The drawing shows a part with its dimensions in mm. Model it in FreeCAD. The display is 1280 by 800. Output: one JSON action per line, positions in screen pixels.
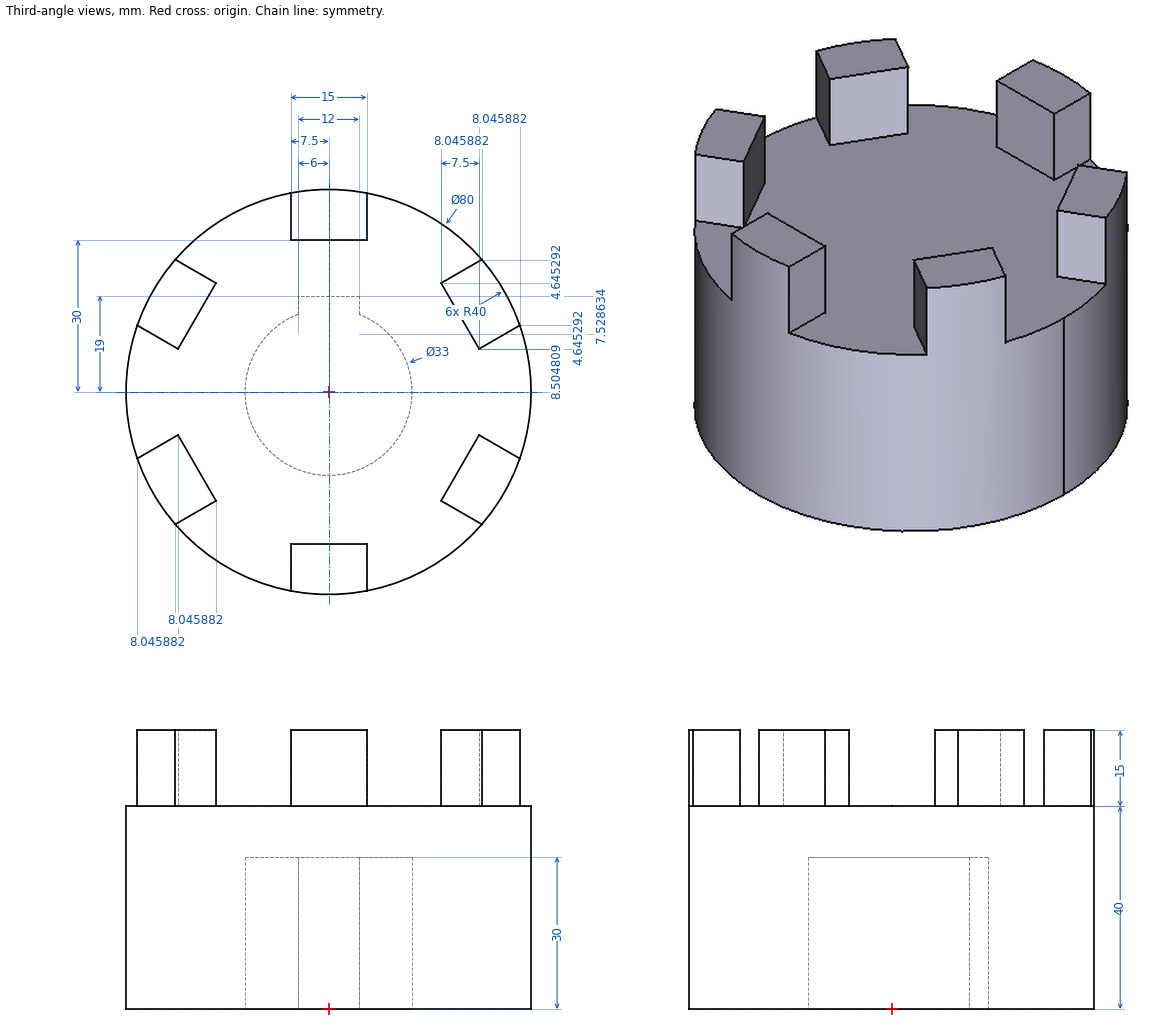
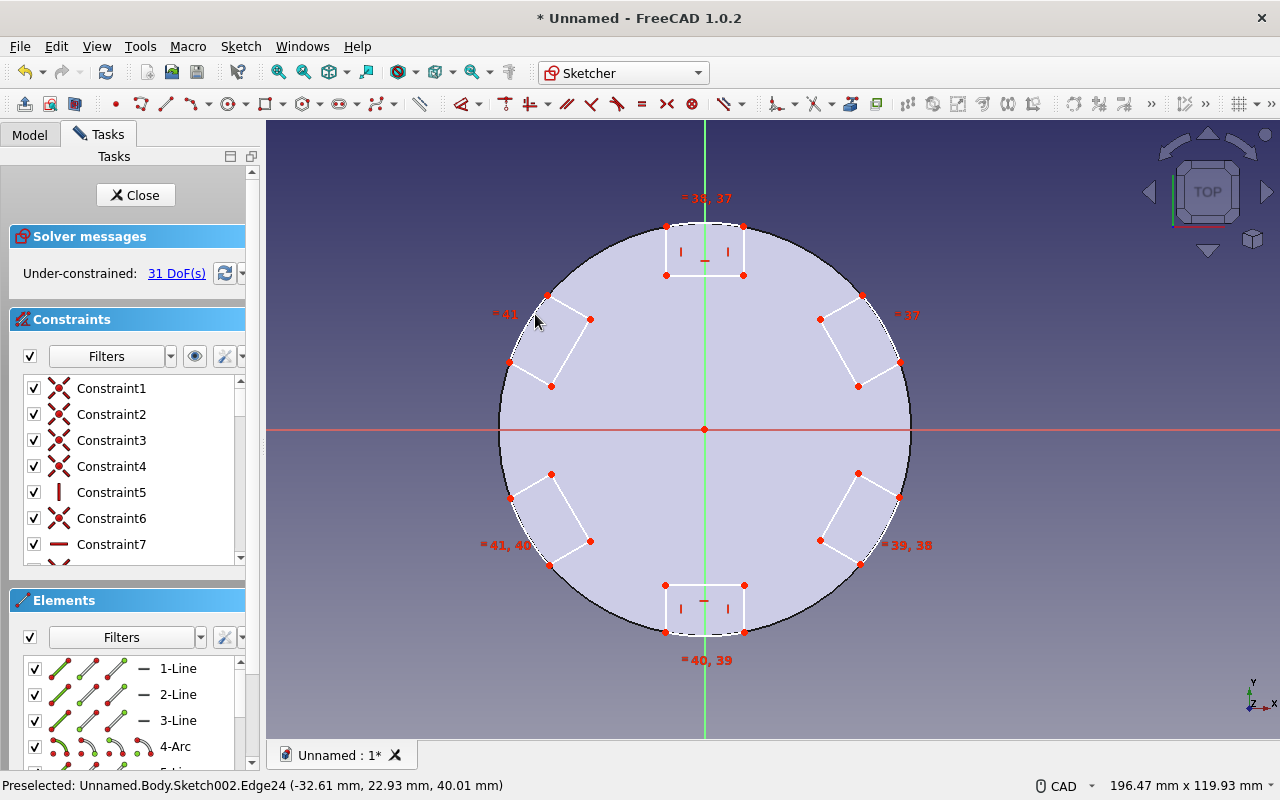
{"action": "left_click", "coordinate": [858, 387]}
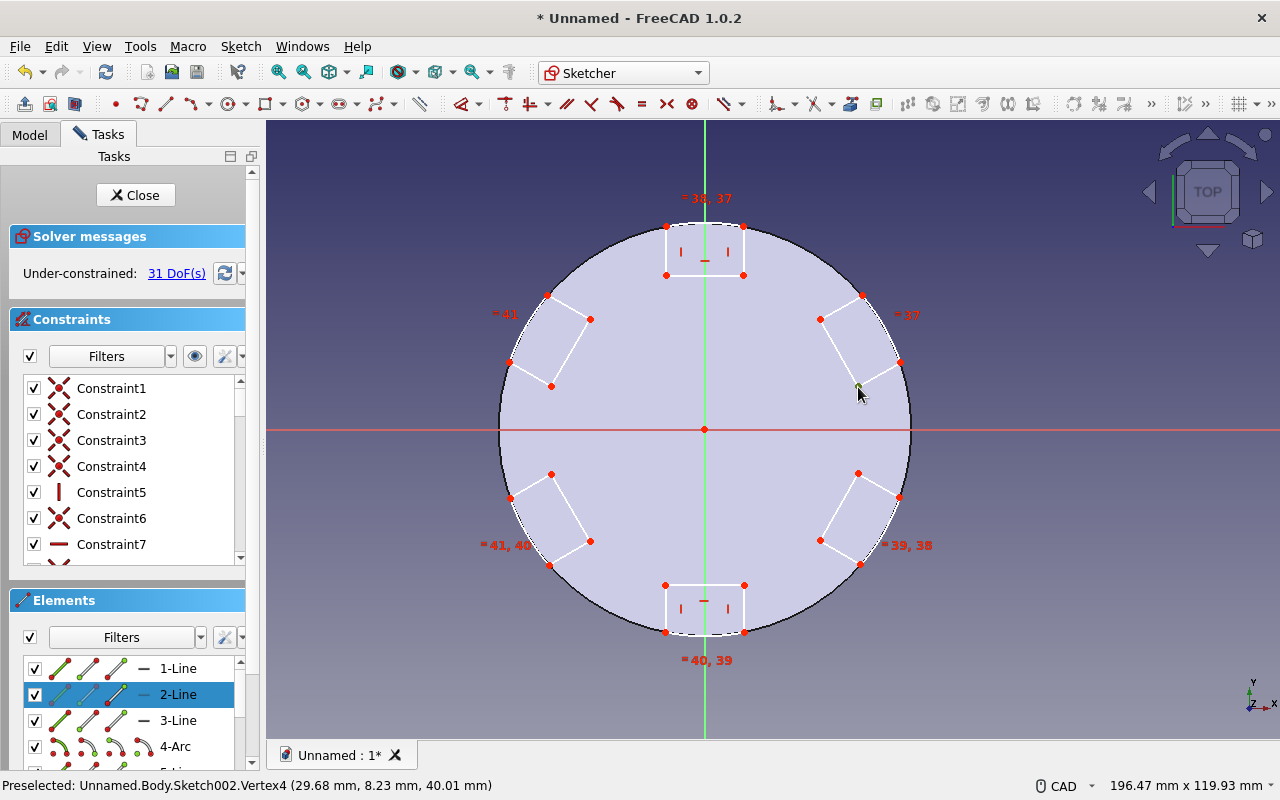
{"action": "left_click", "coordinate": [858, 474]}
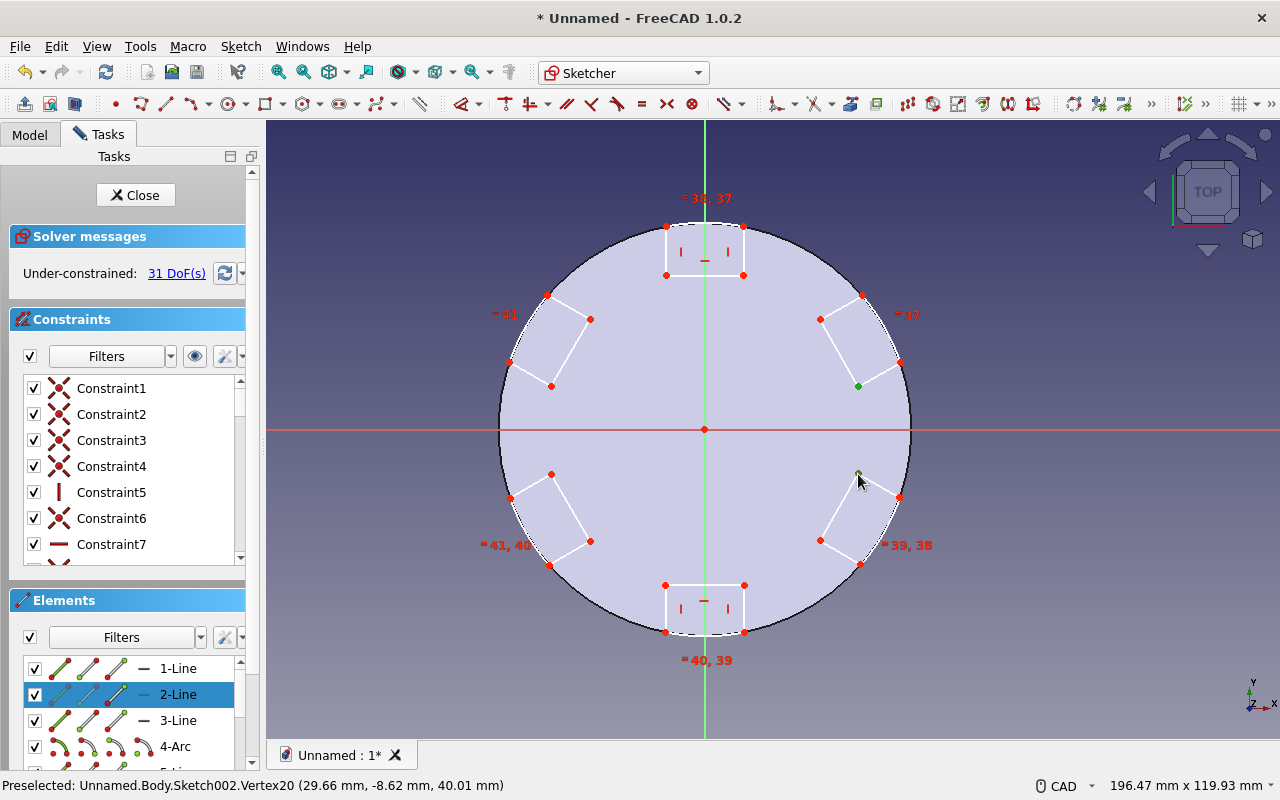
{"action": "left_click", "coordinate": [353, 429]}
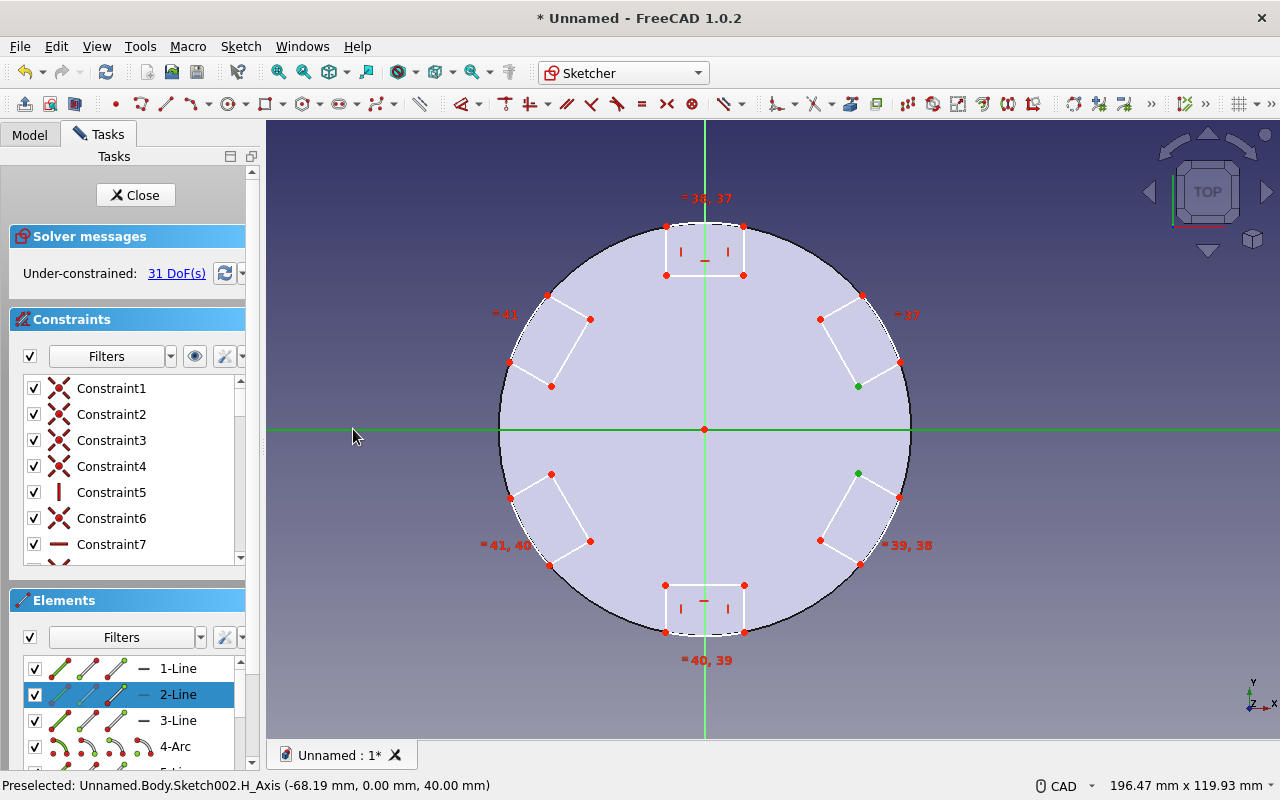
{"action": "left_click", "coordinate": [667, 104]}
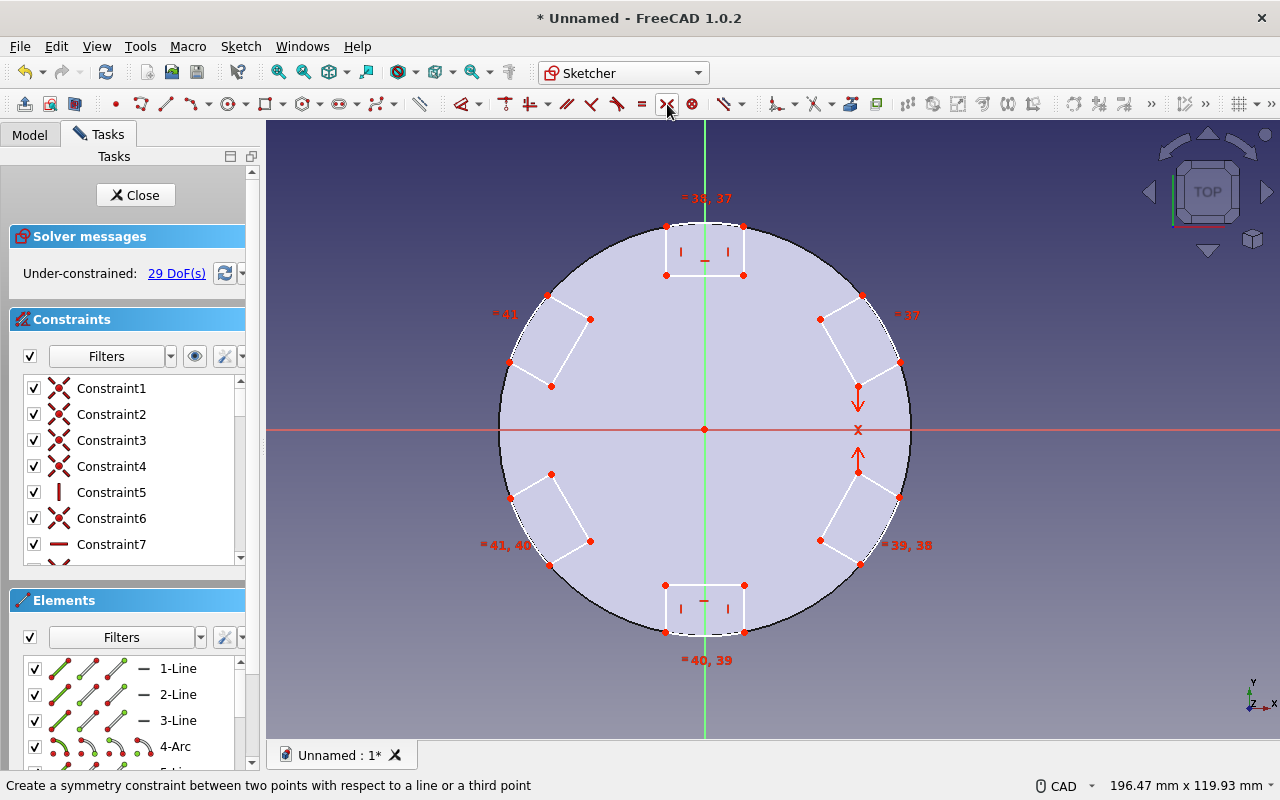
{"action": "left_click", "coordinate": [820, 320]}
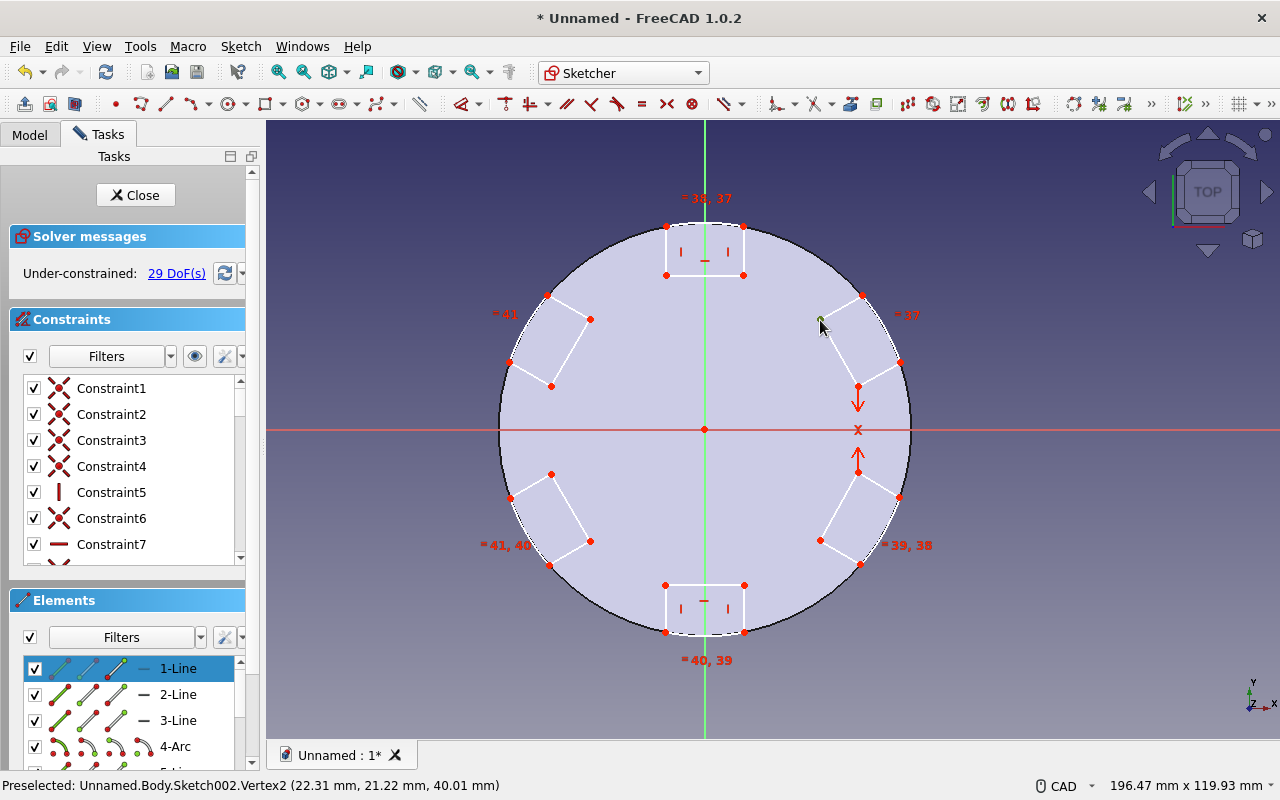
{"action": "left_click", "coordinate": [820, 541]}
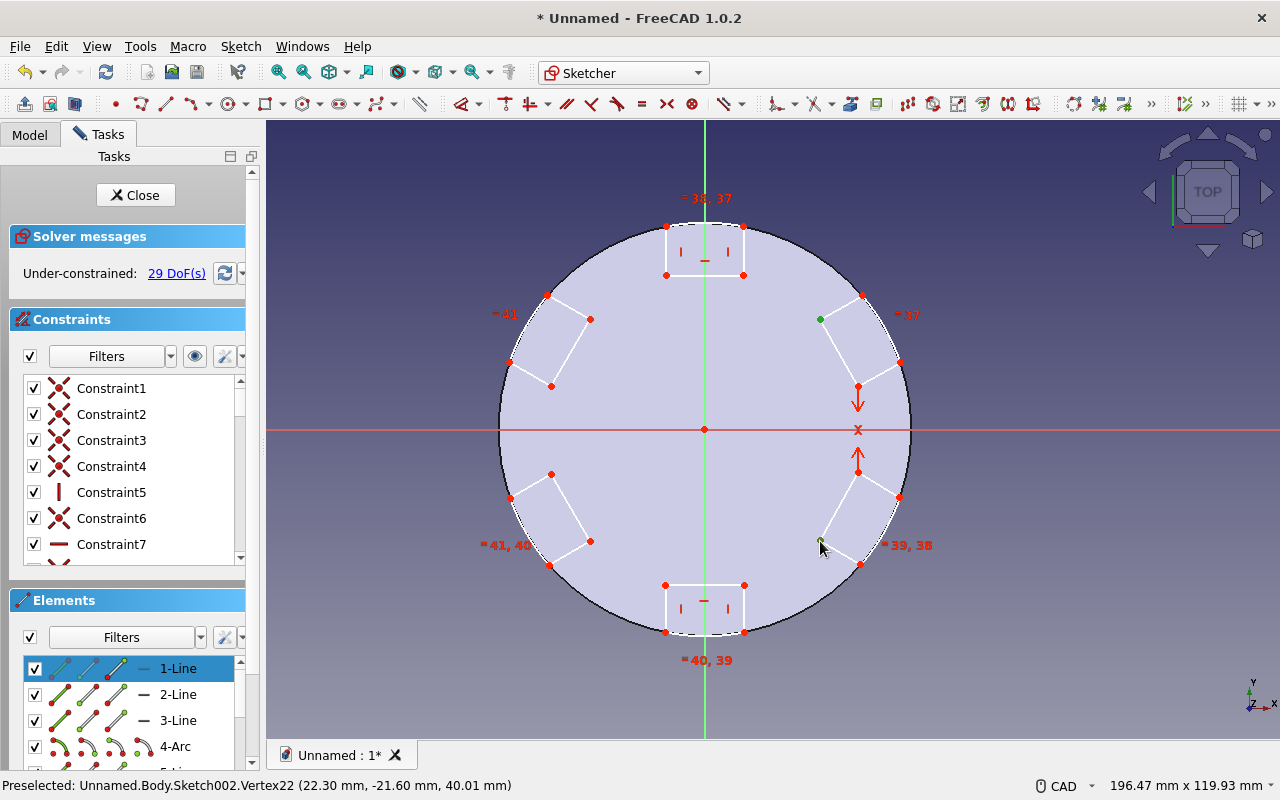
{"action": "left_click", "coordinate": [353, 429]}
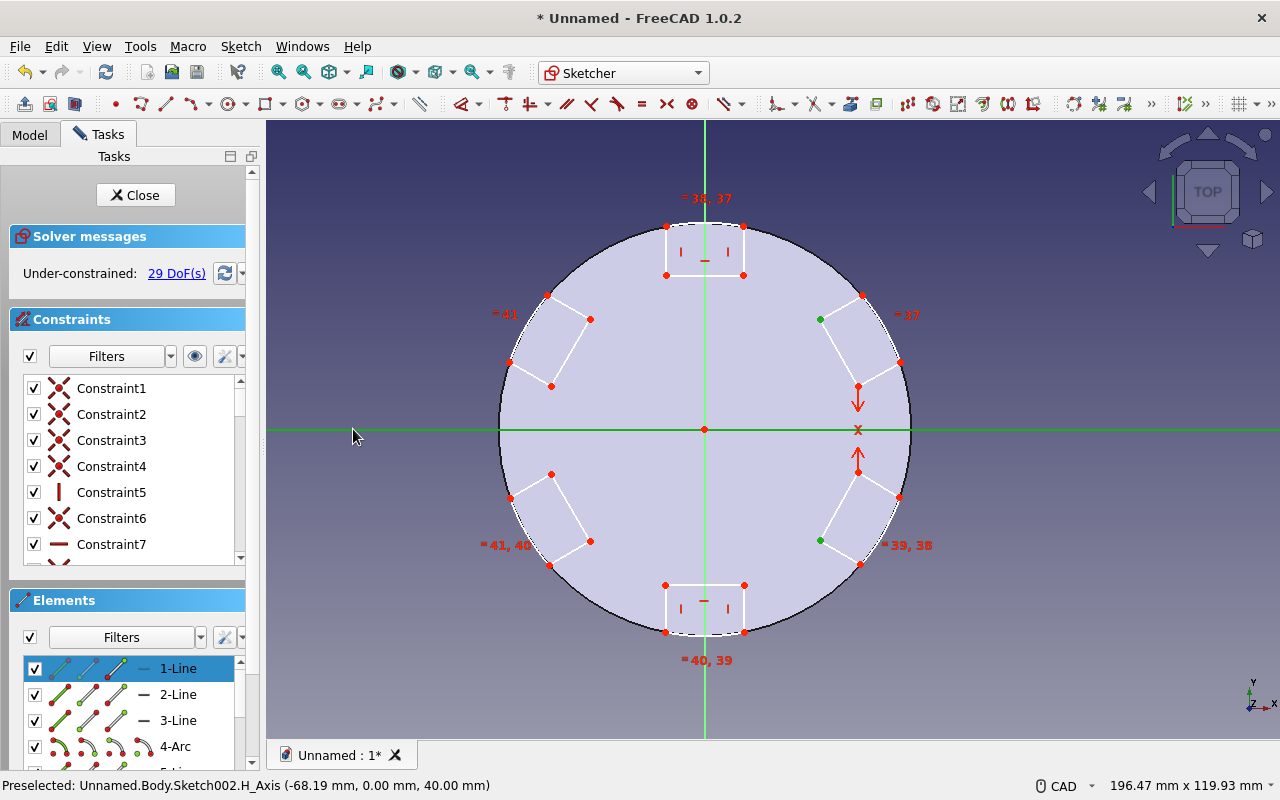
{"action": "key", "text": "s"}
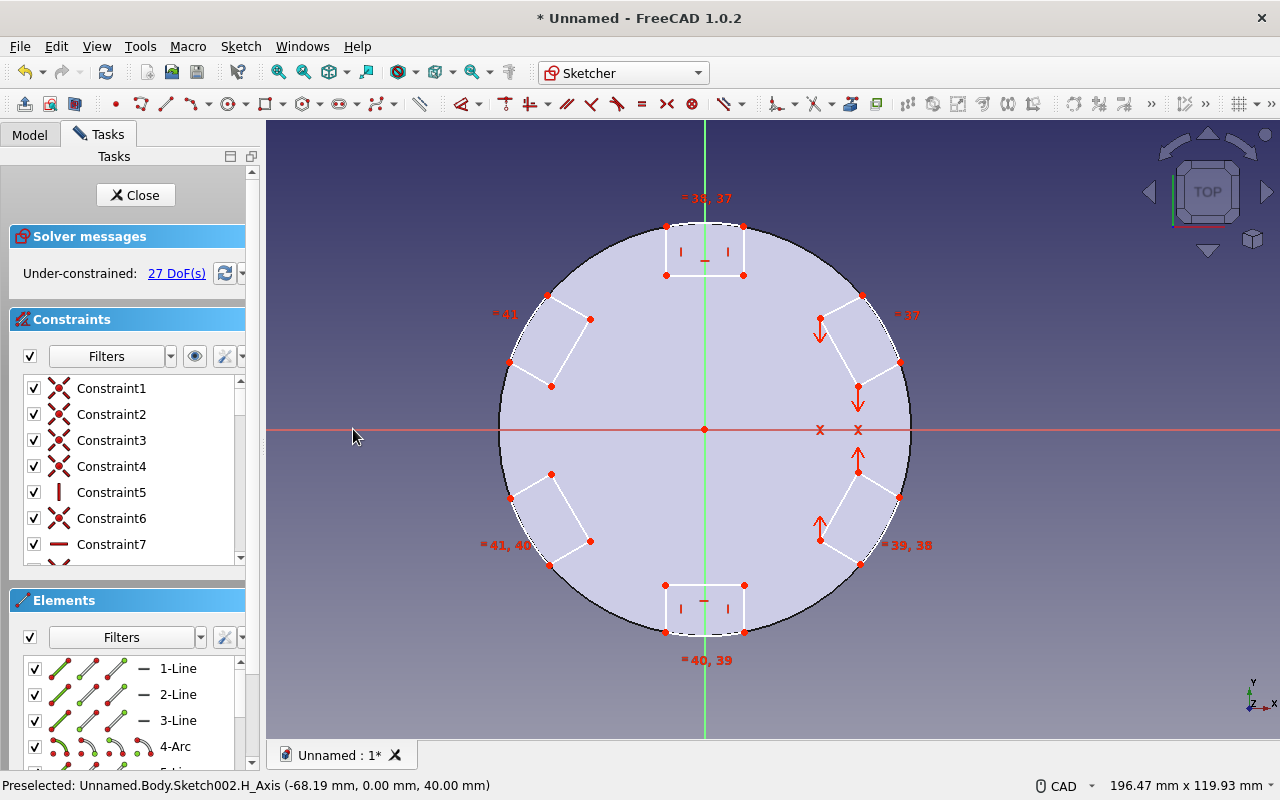
{"action": "left_click", "coordinate": [744, 276]}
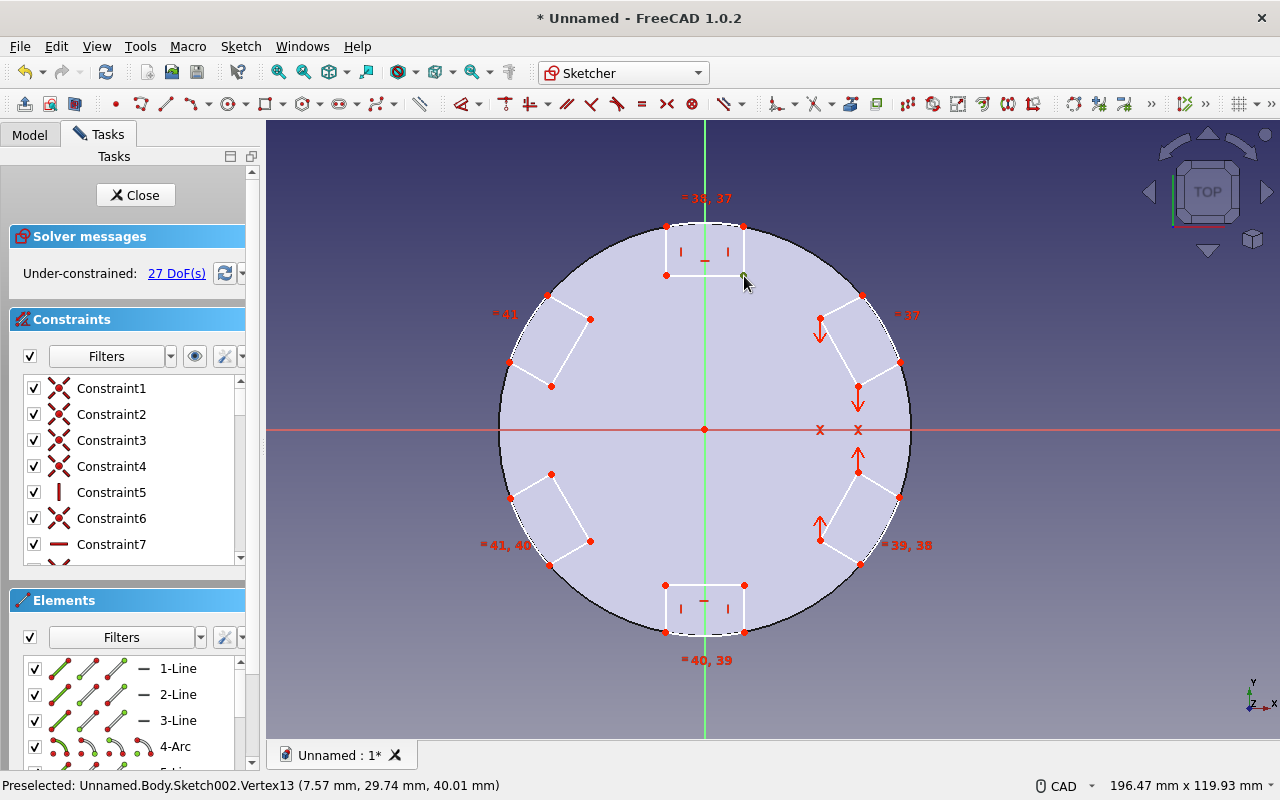
{"action": "left_click", "coordinate": [744, 585]}